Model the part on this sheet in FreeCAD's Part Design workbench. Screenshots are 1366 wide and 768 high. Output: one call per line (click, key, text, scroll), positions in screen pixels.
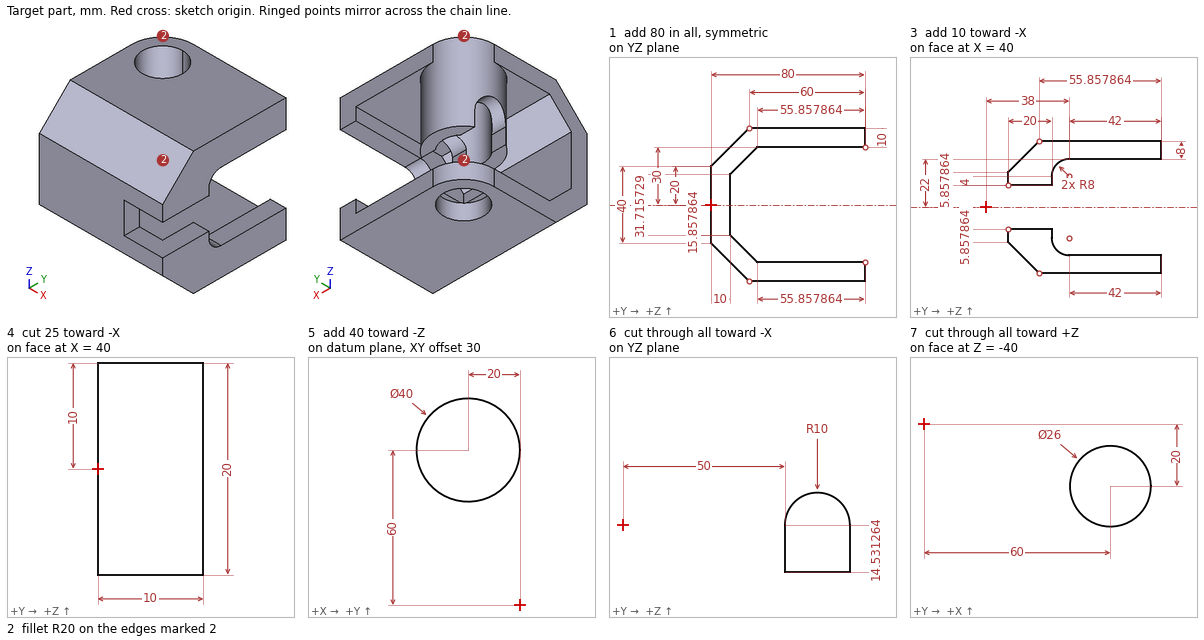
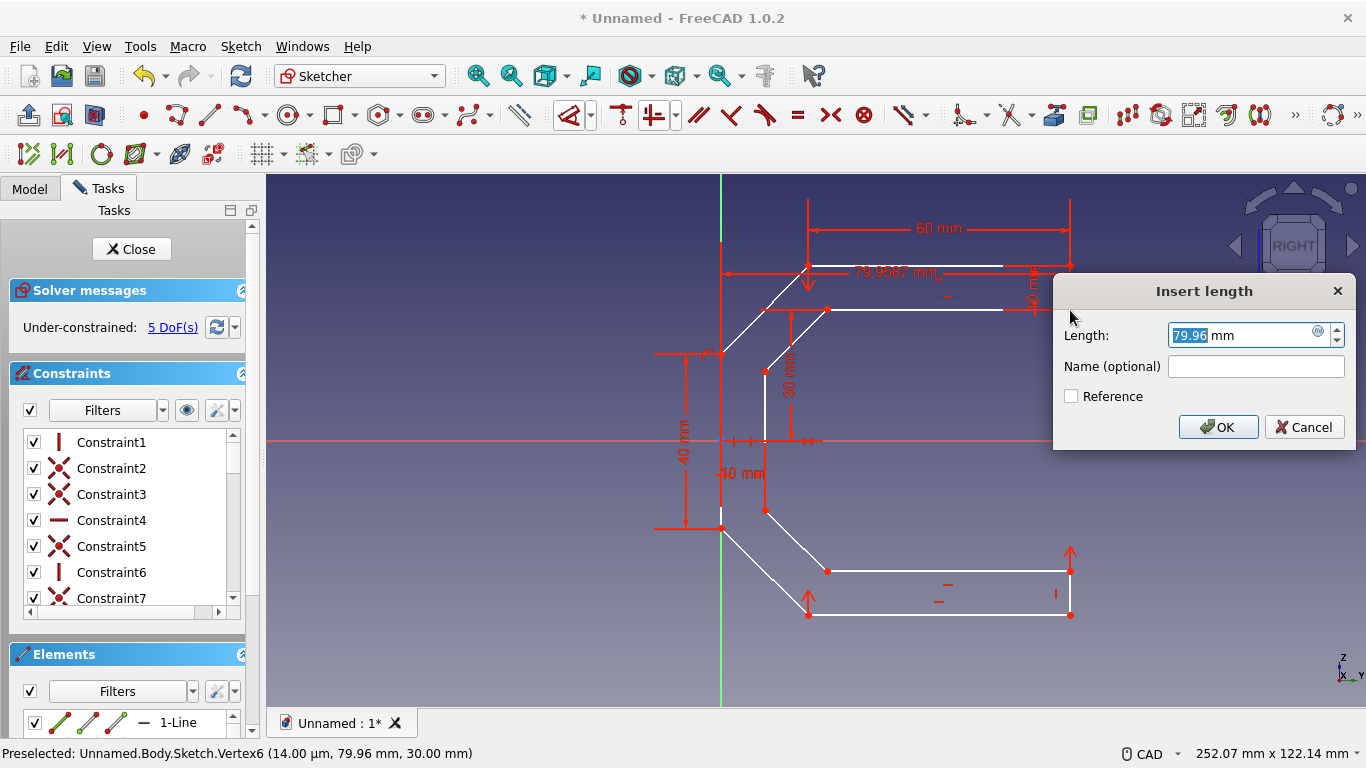
text(80)
key(Return)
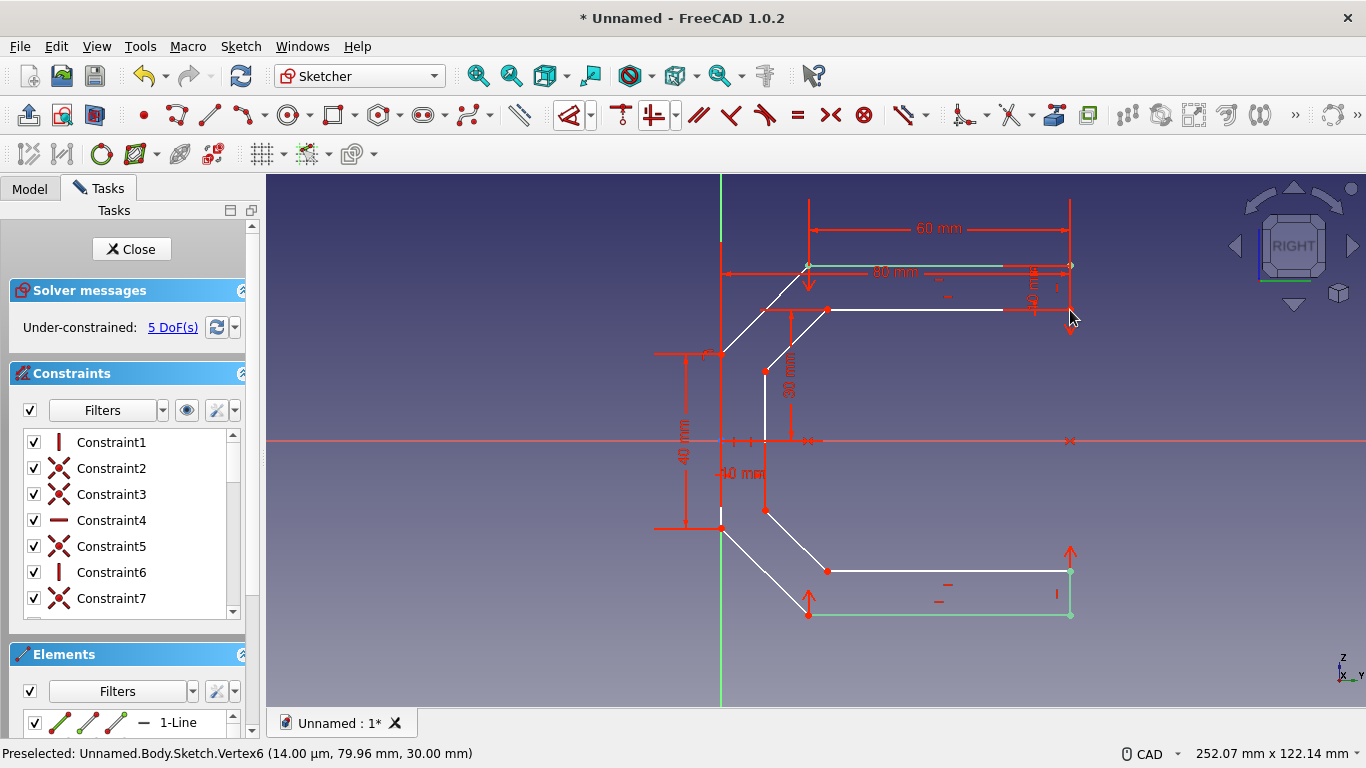
click(721, 354)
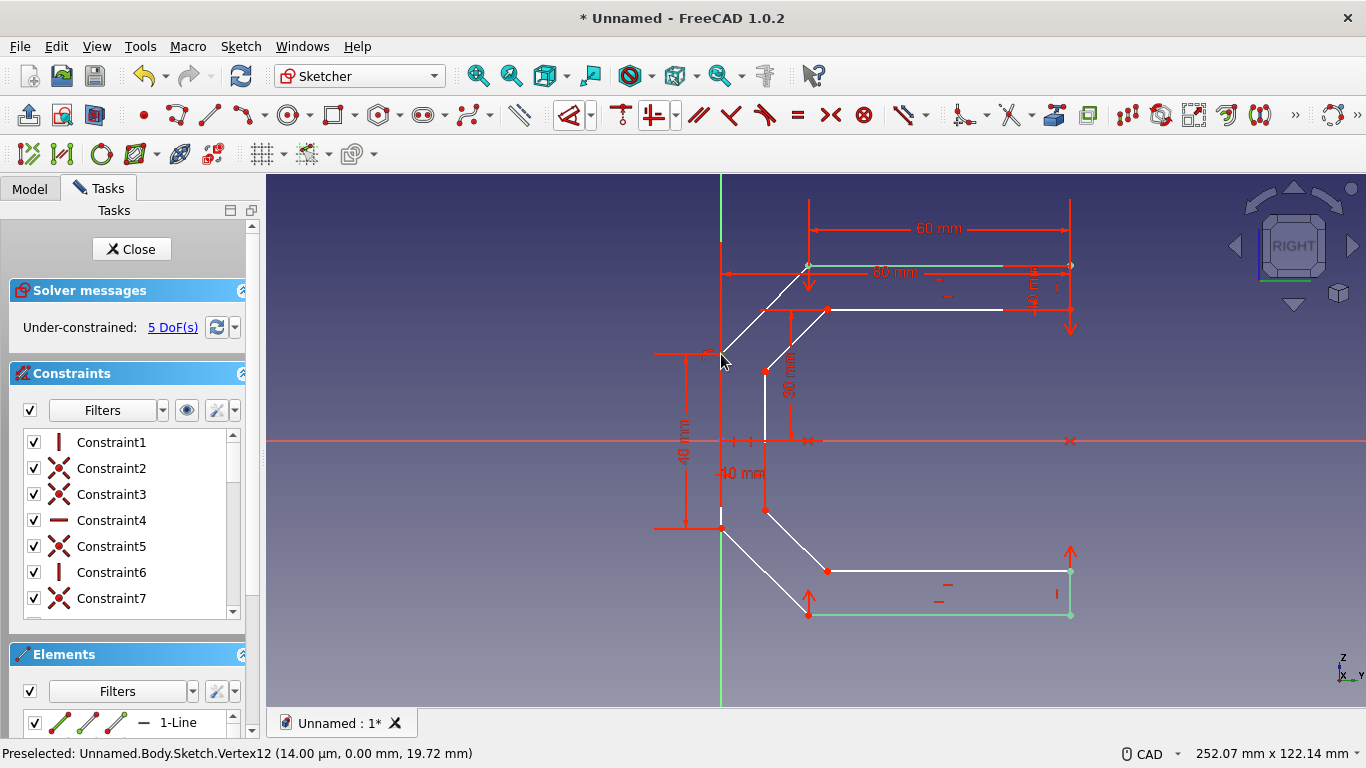
click(590, 116)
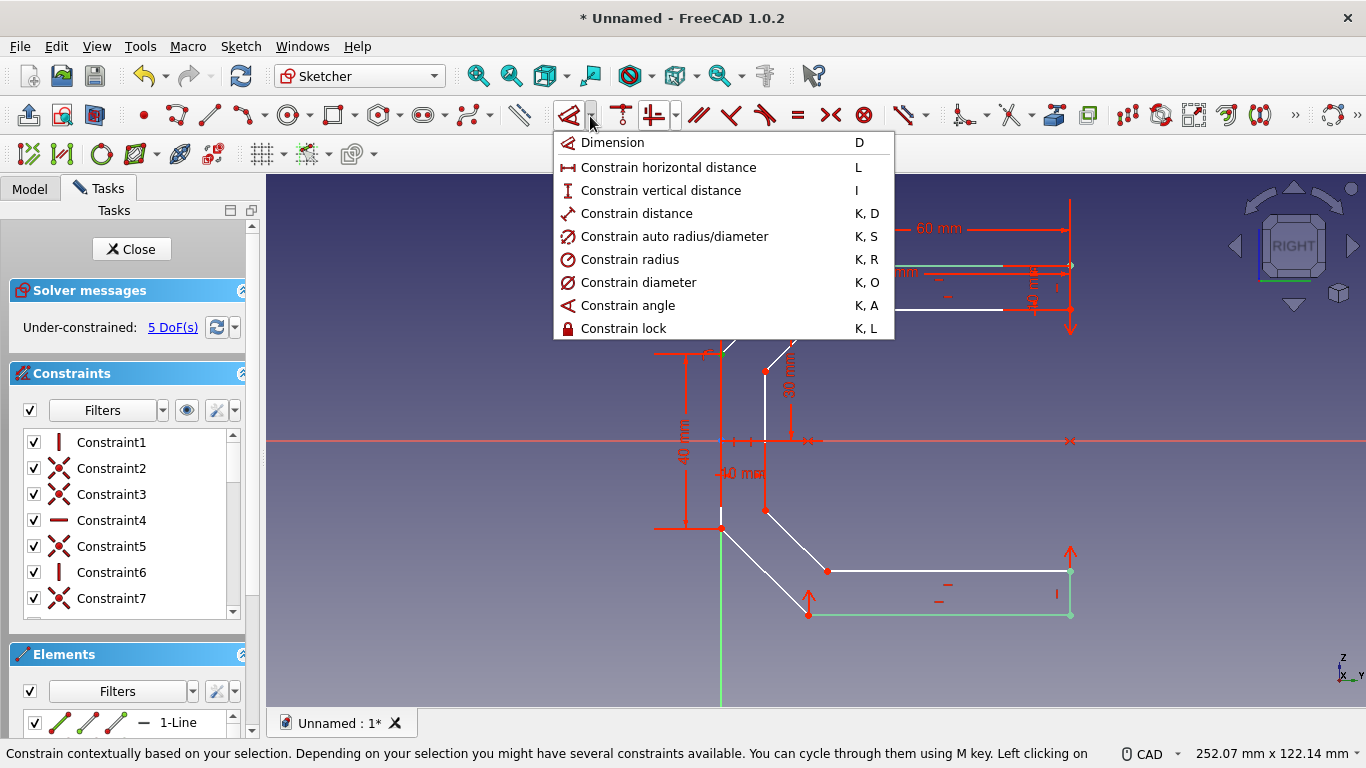
click(724, 190)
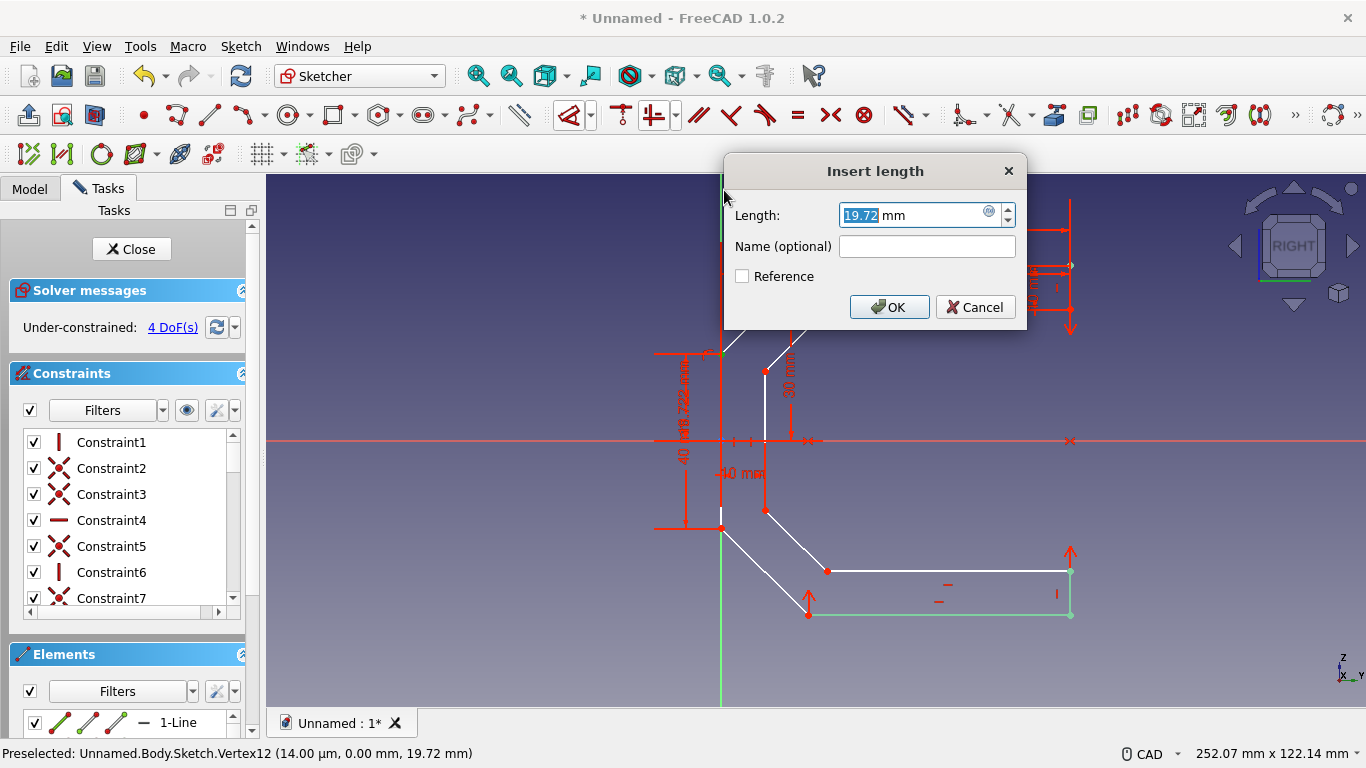
text(20)
key(Return)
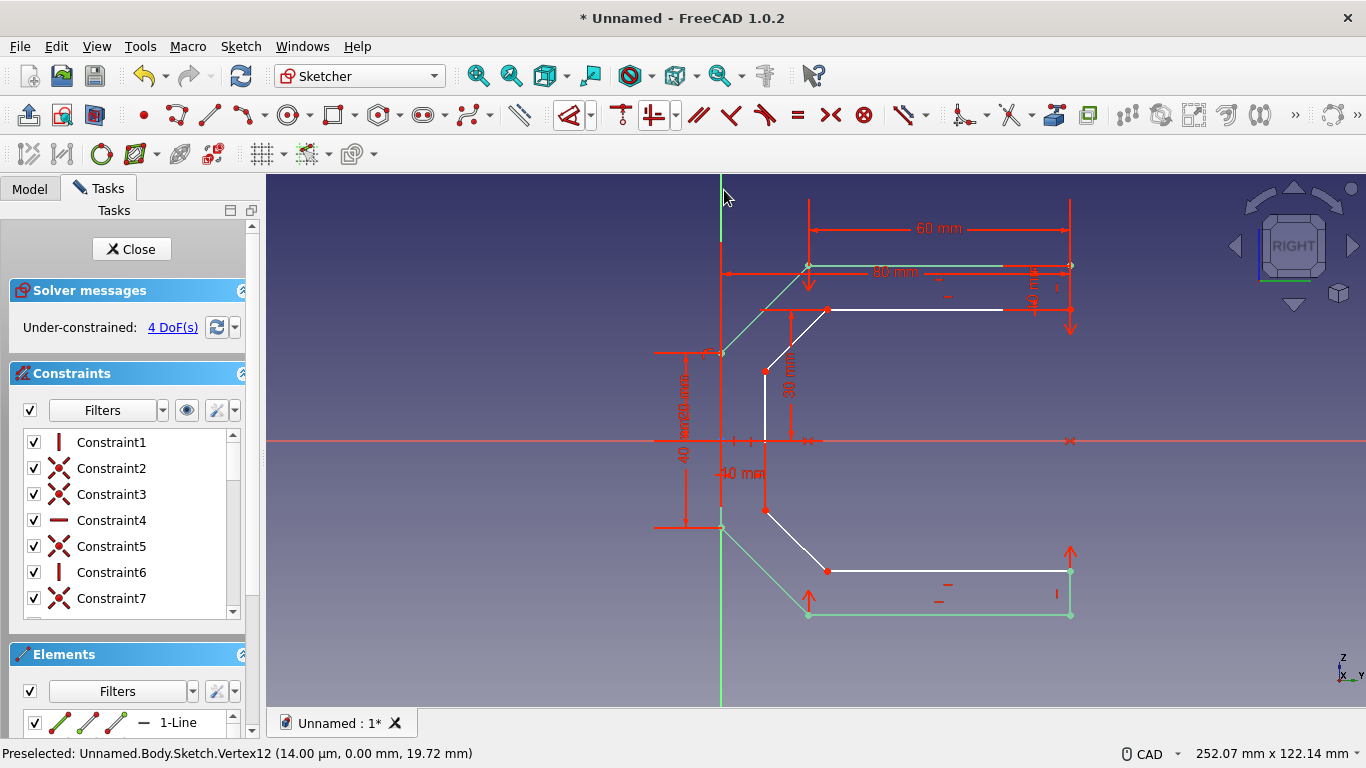
click(765, 414)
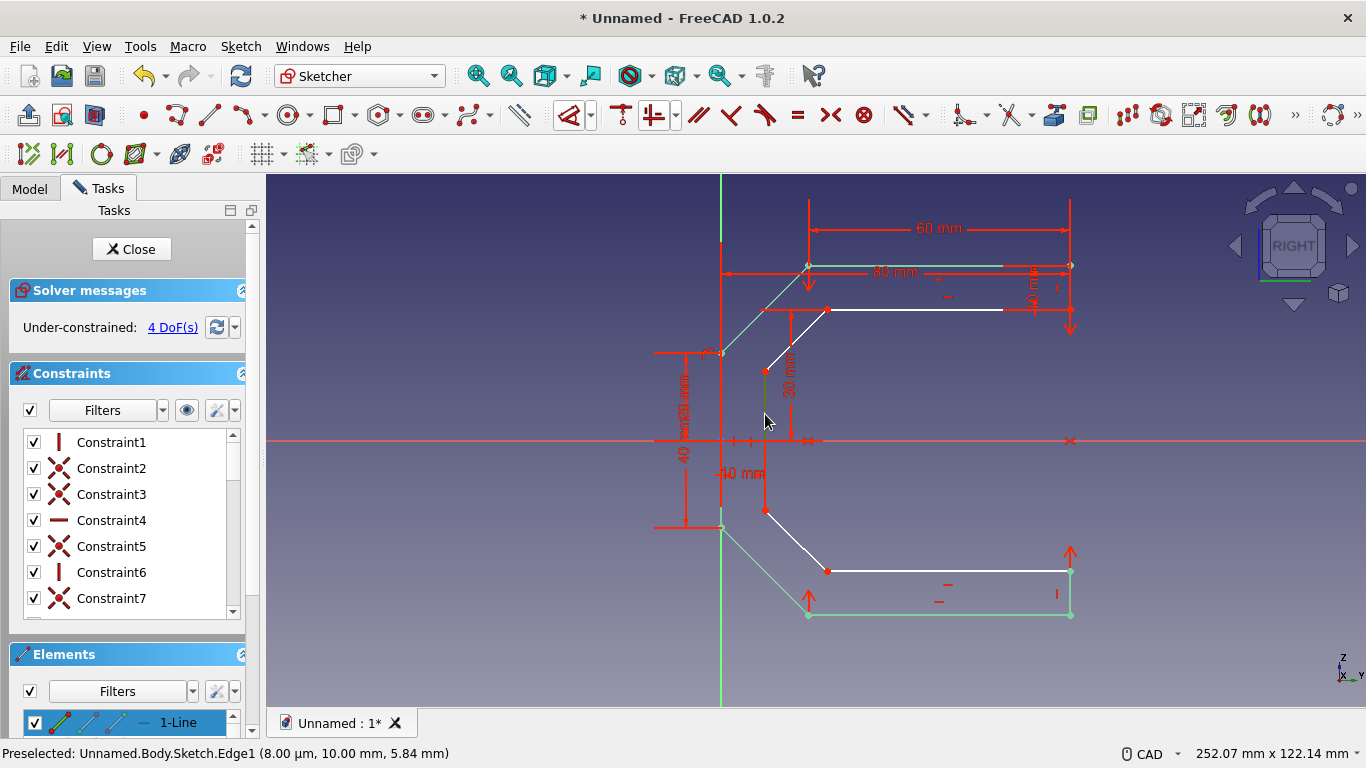
click(590, 116)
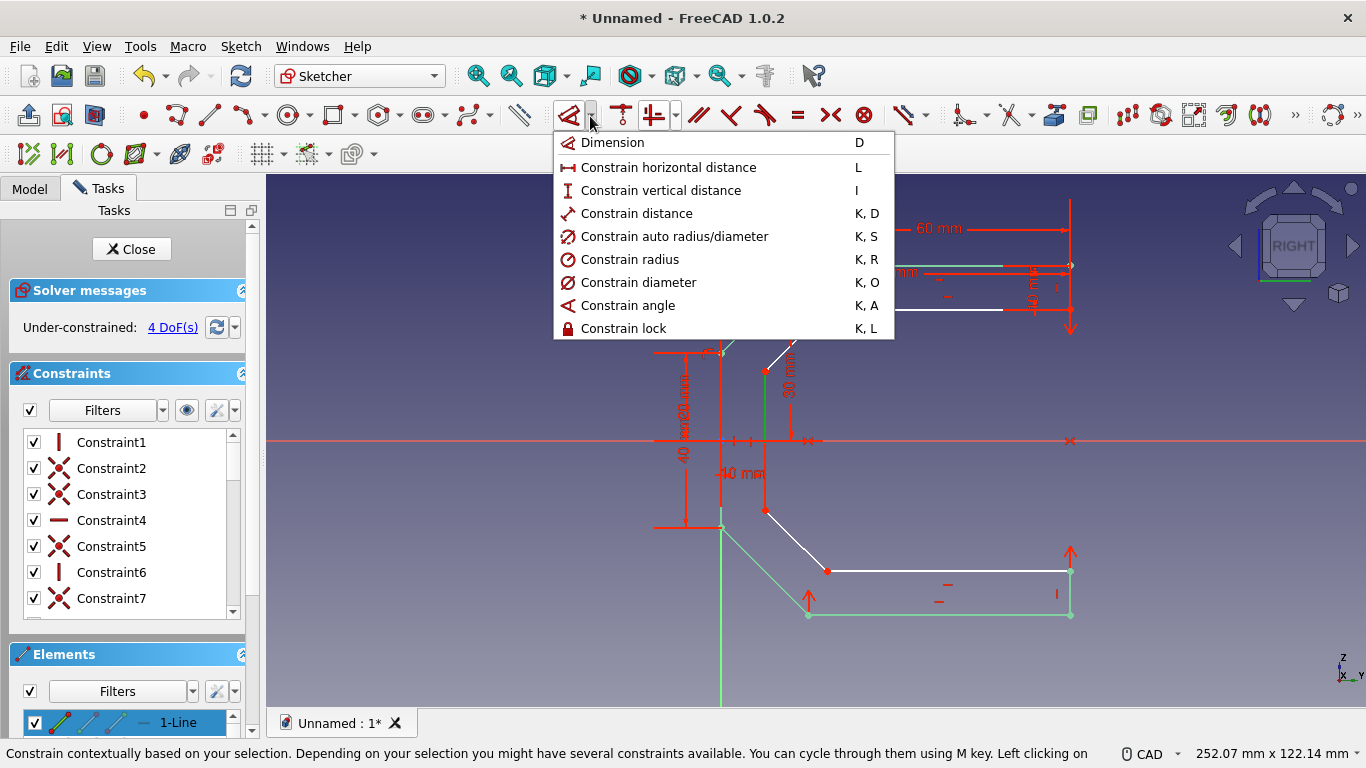
click(724, 190)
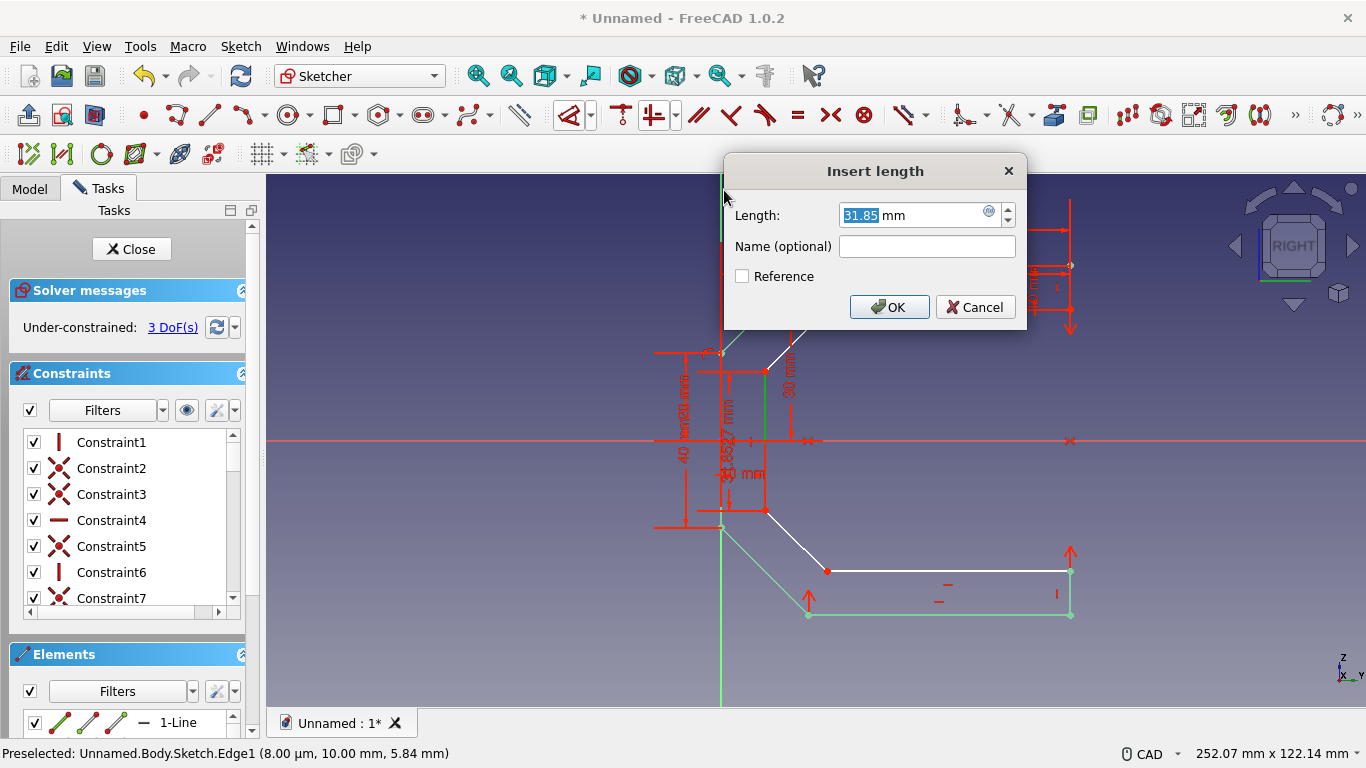
text(31.715729)
key(Return)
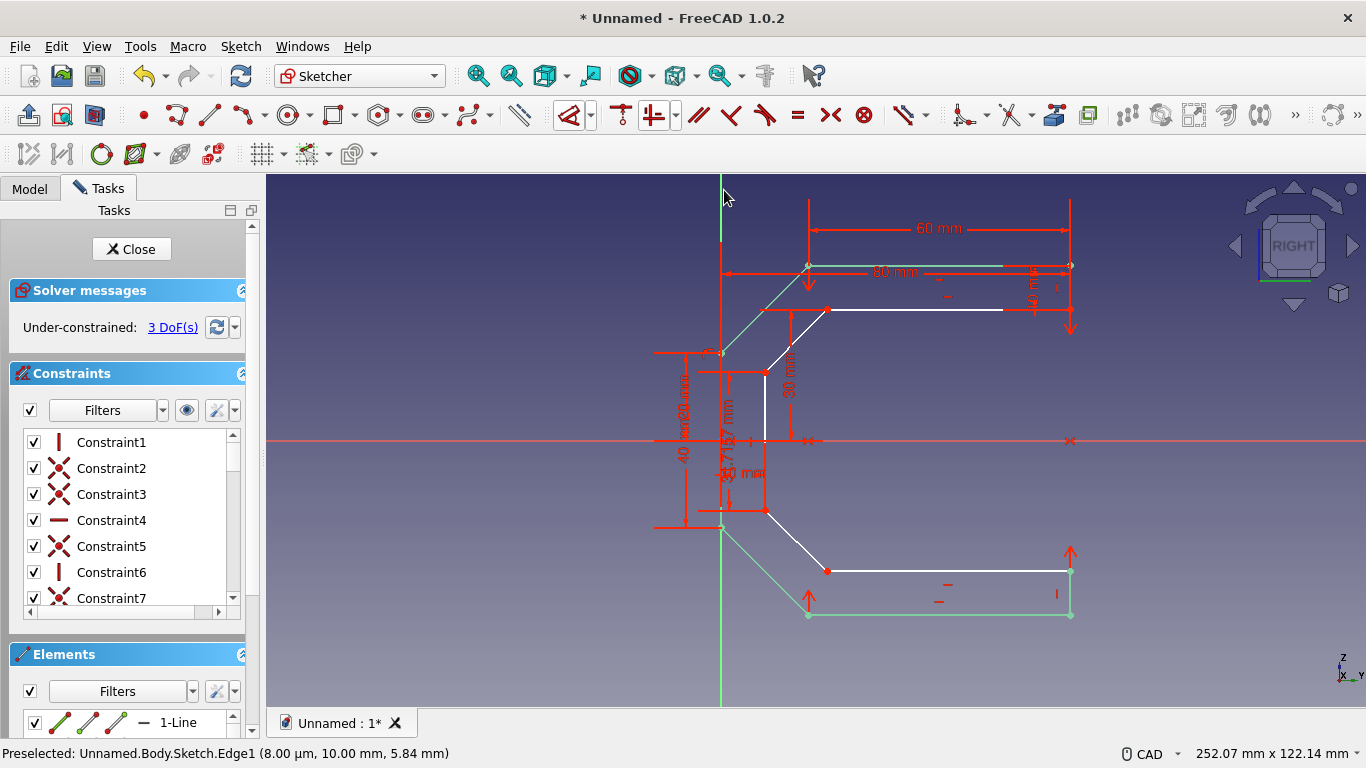
click(900, 310)